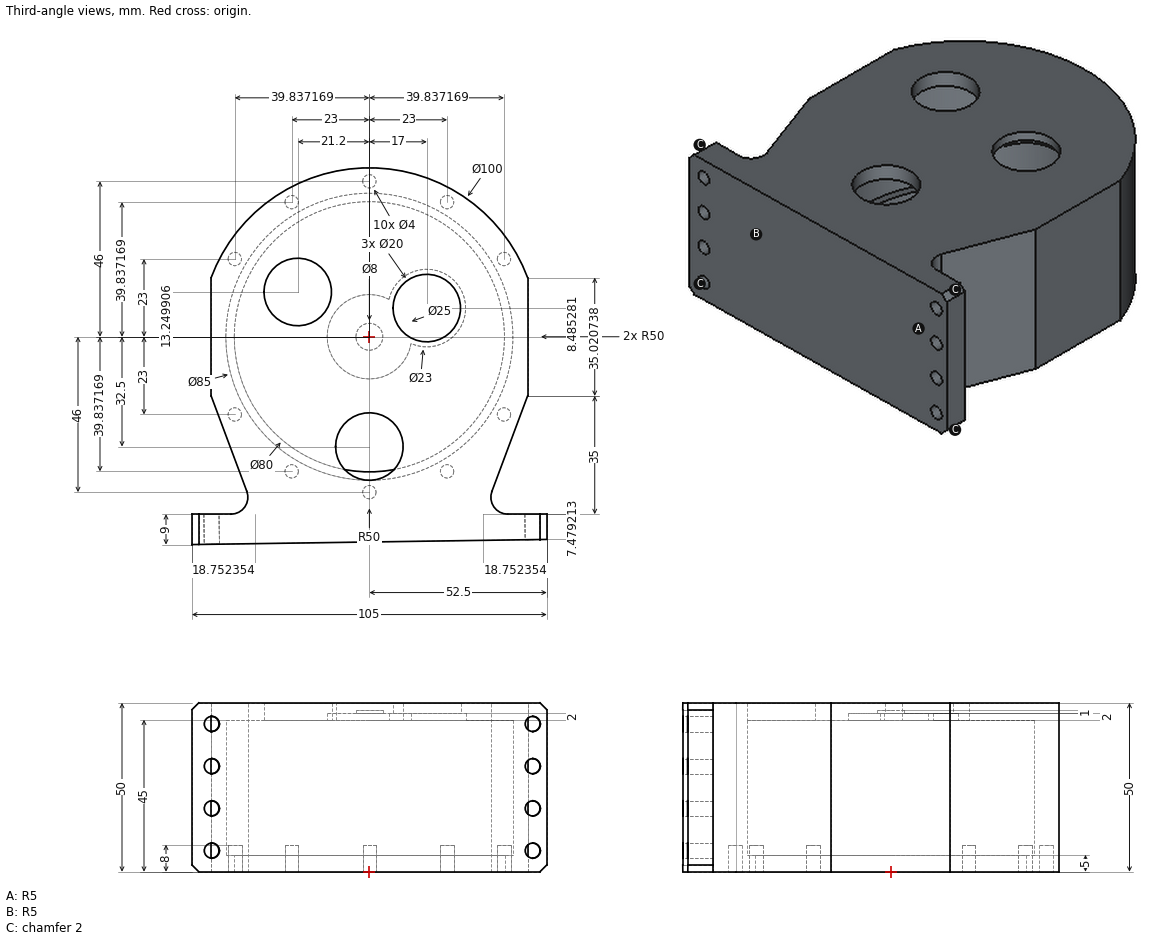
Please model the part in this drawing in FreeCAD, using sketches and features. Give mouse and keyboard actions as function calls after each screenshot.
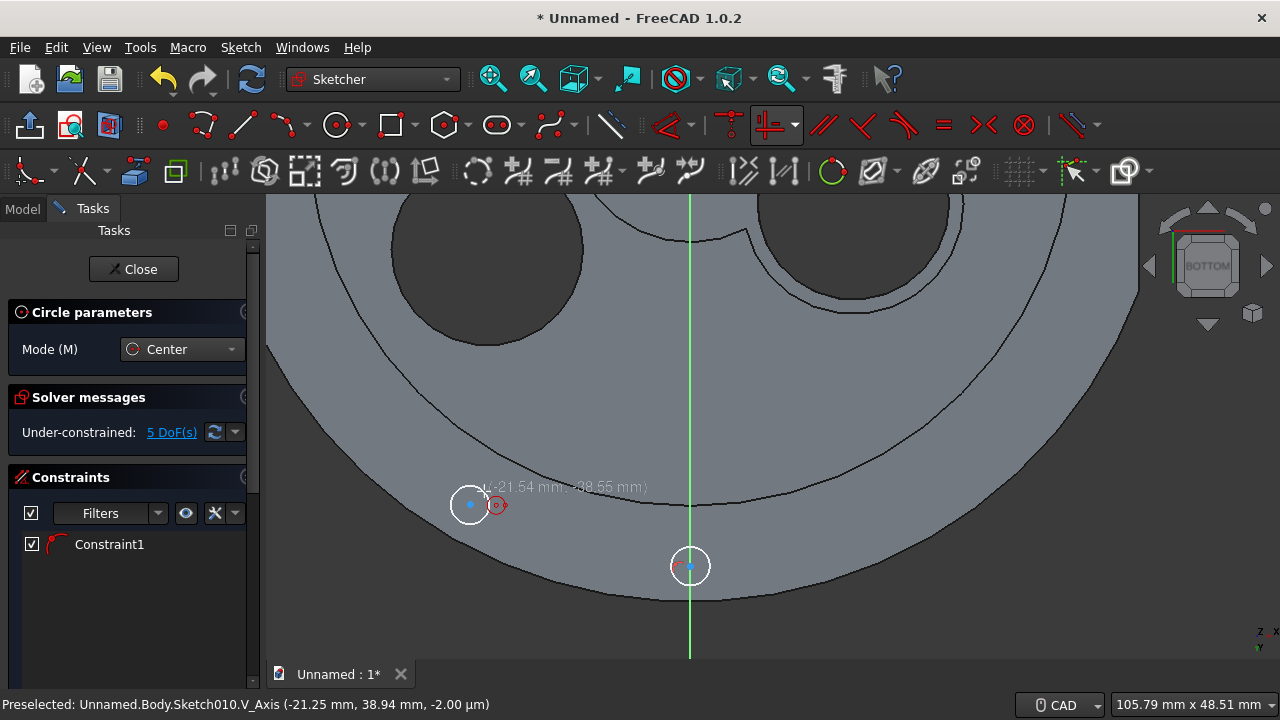
click(309, 343)
click(322, 329)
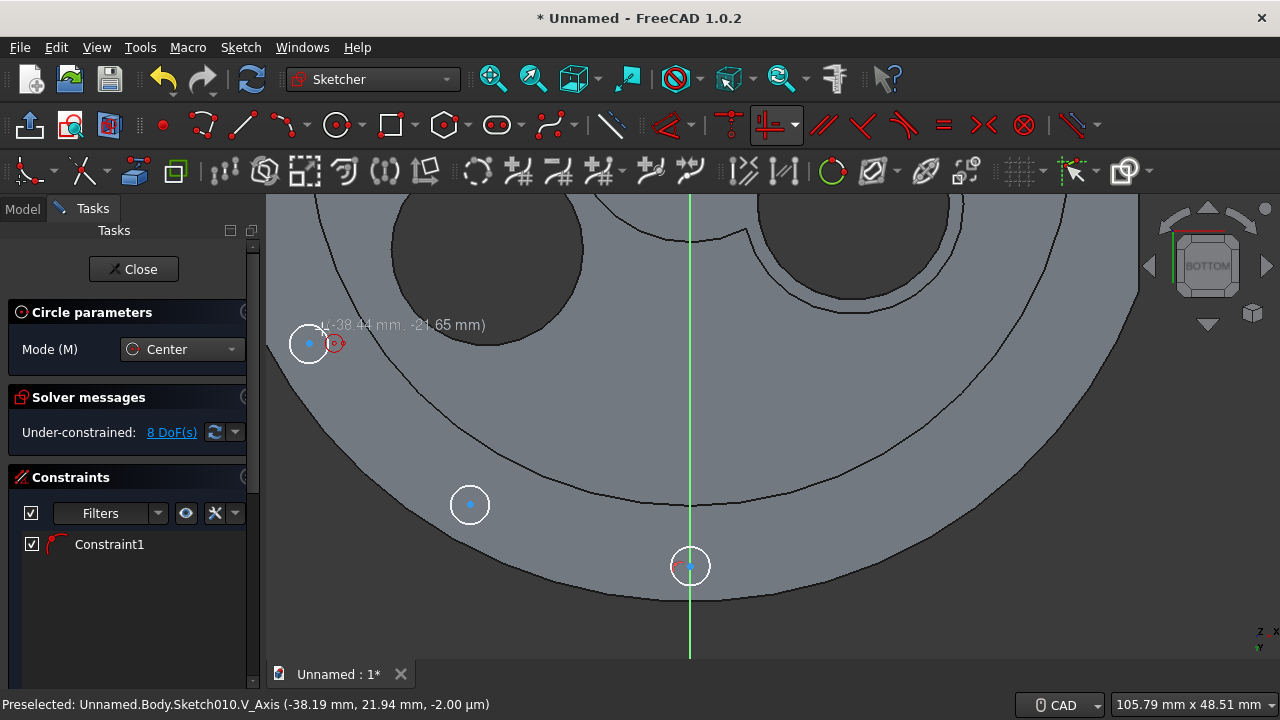
click(911, 504)
click(925, 491)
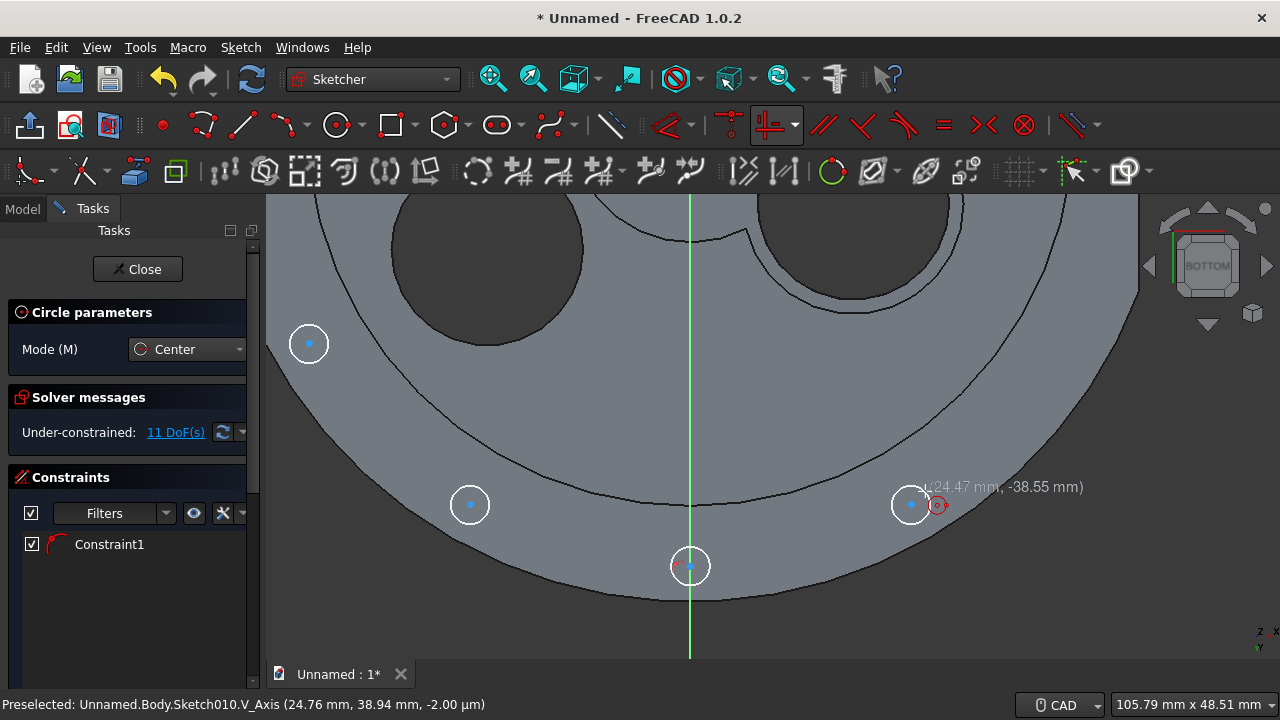
click(1072, 343)
click(1086, 329)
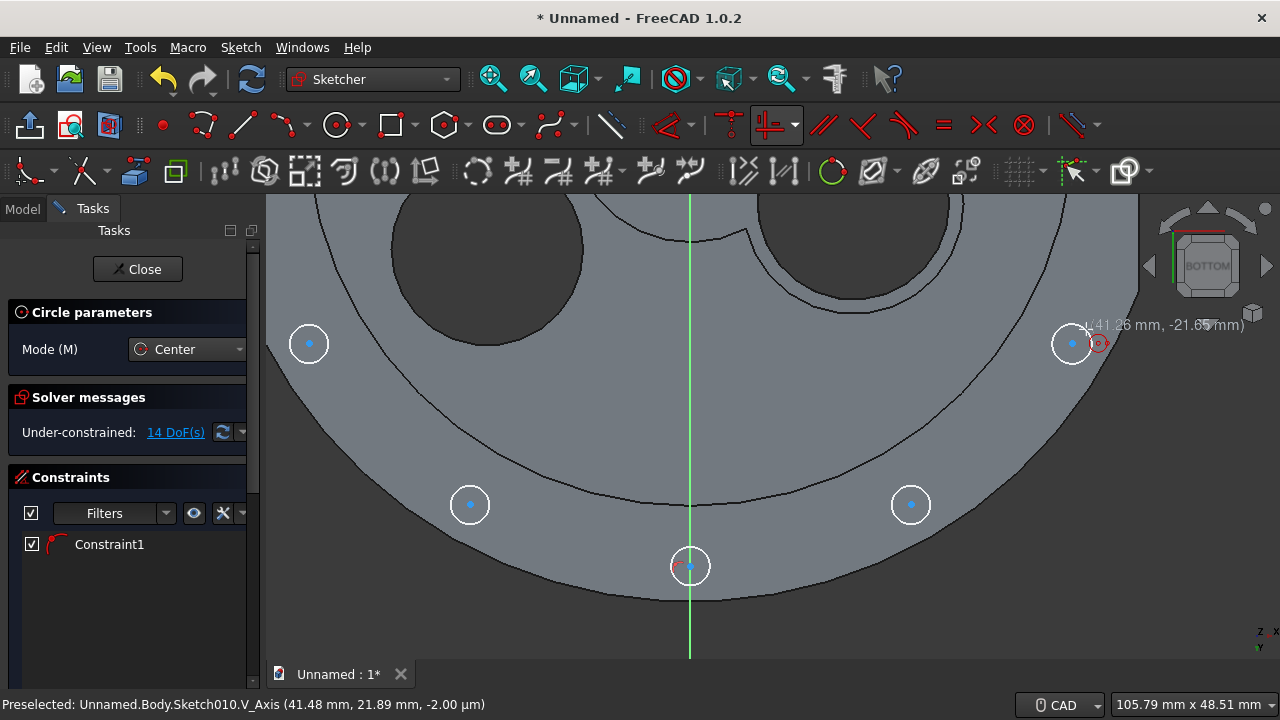
scroll(711, 558, down, 6)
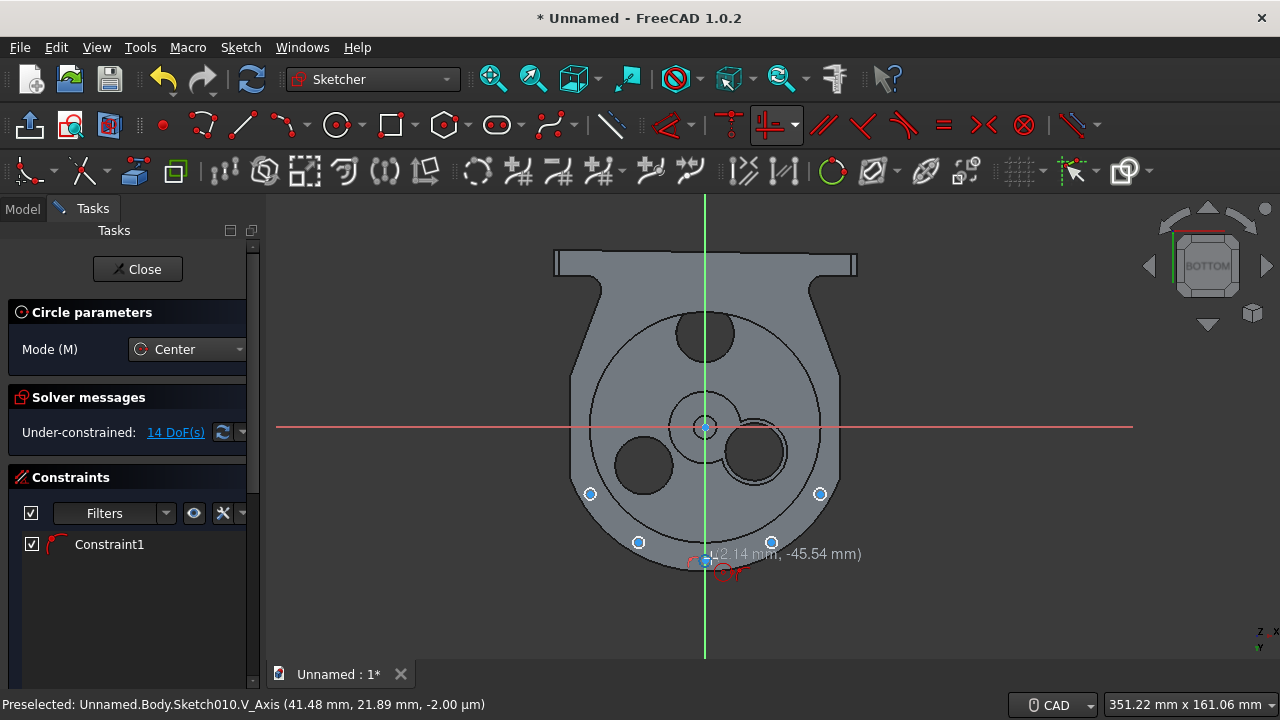
scroll(590, 361, up, 7)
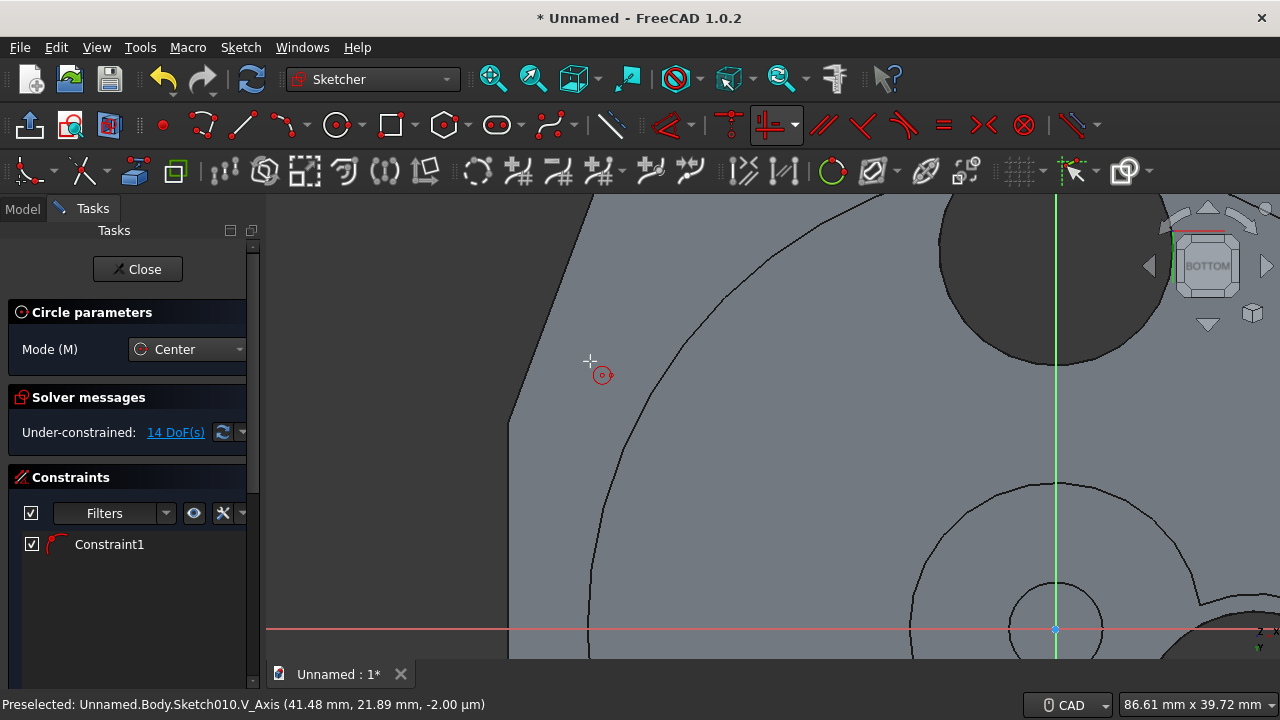
scroll(589, 360, down, 7)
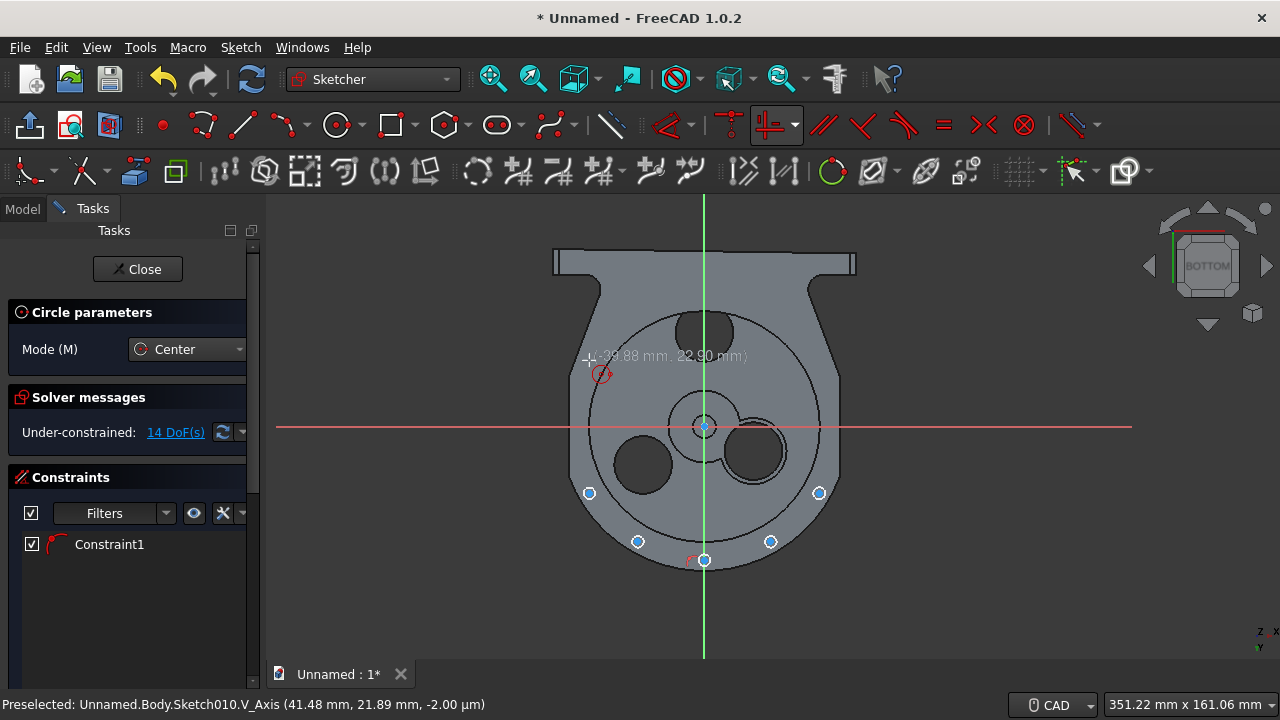
click(589, 360)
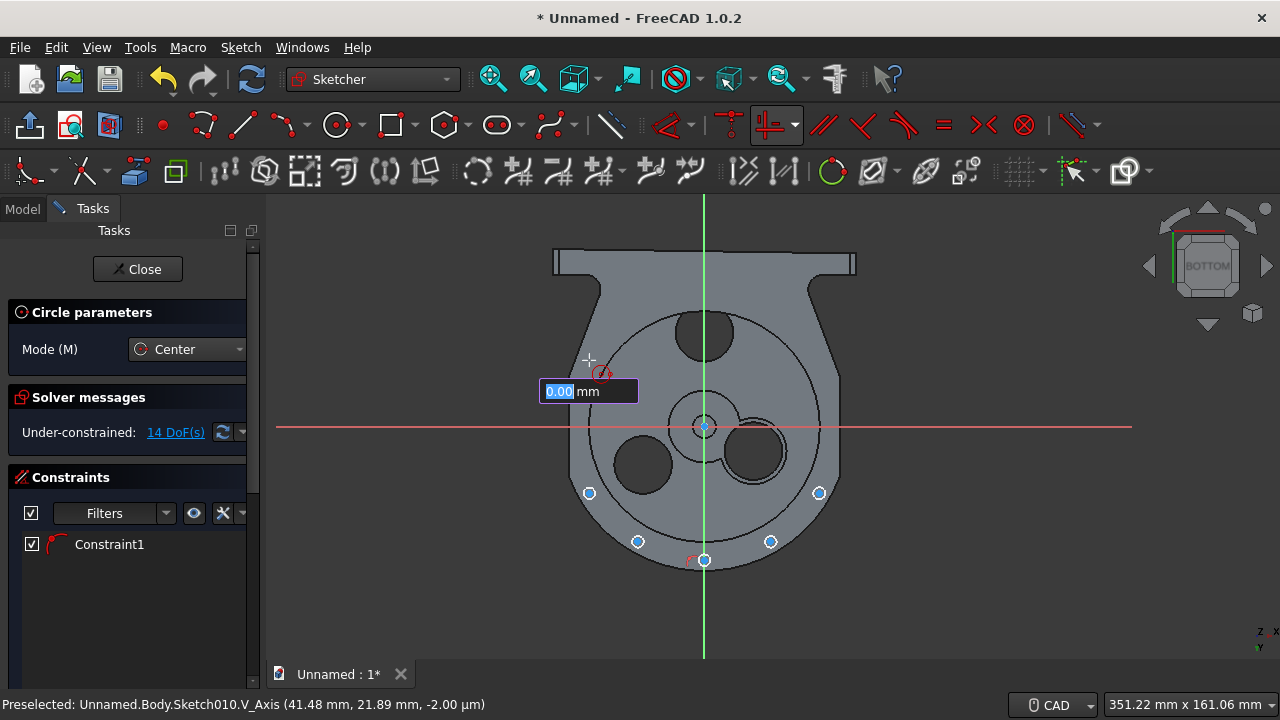
scroll(593, 356, up, 6)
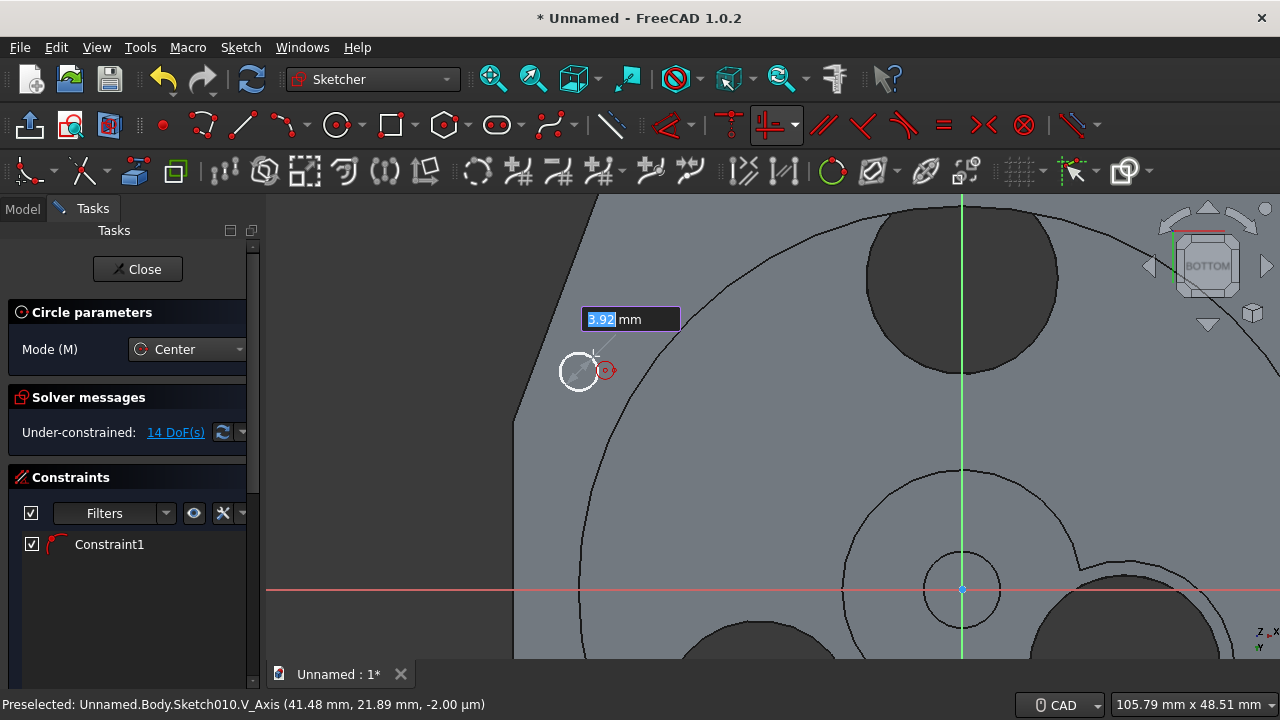
click(594, 356)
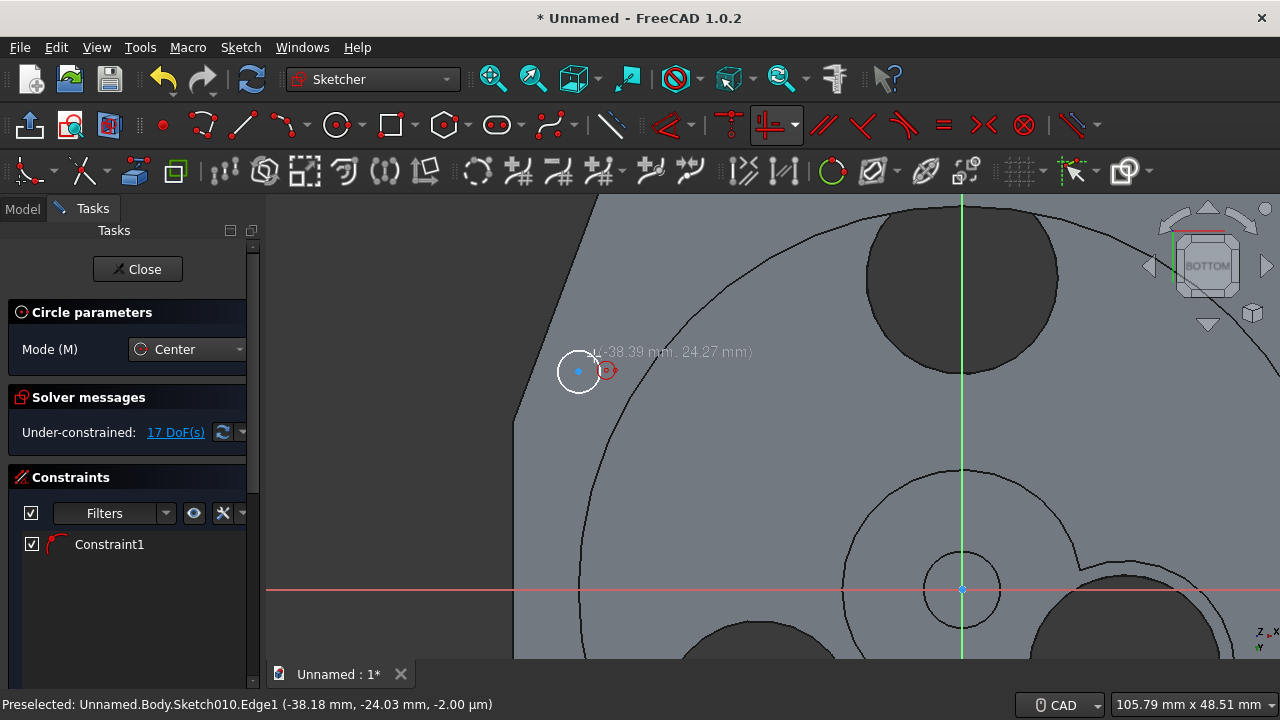
scroll(594, 356, down, 6)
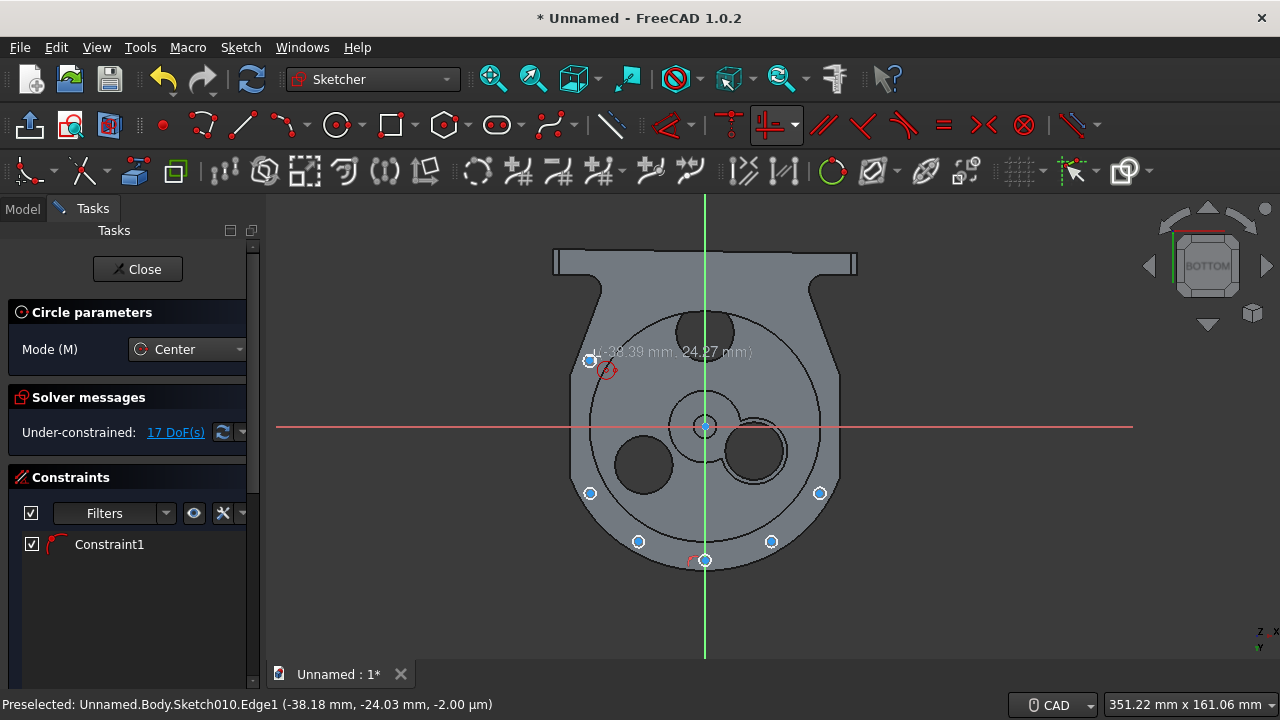
scroll(639, 312, up, 7)